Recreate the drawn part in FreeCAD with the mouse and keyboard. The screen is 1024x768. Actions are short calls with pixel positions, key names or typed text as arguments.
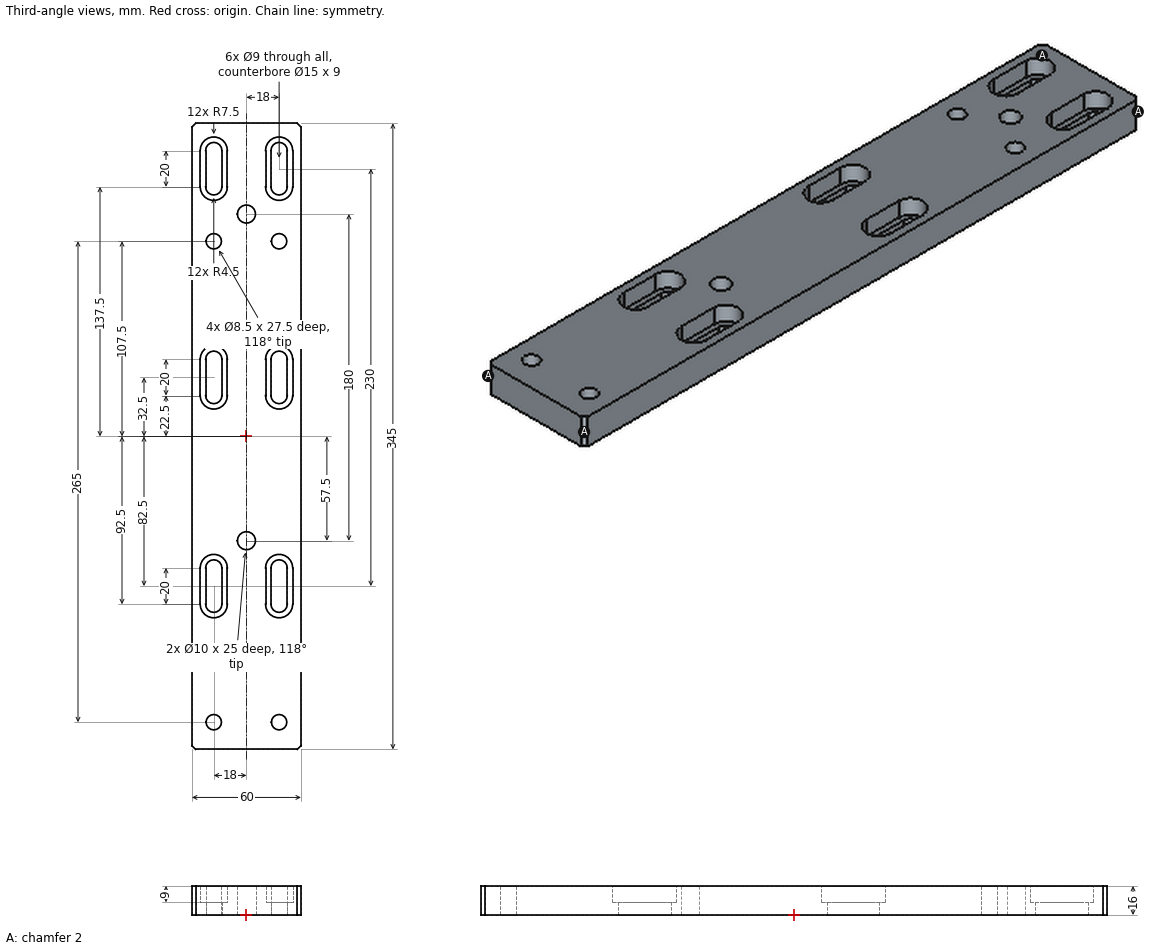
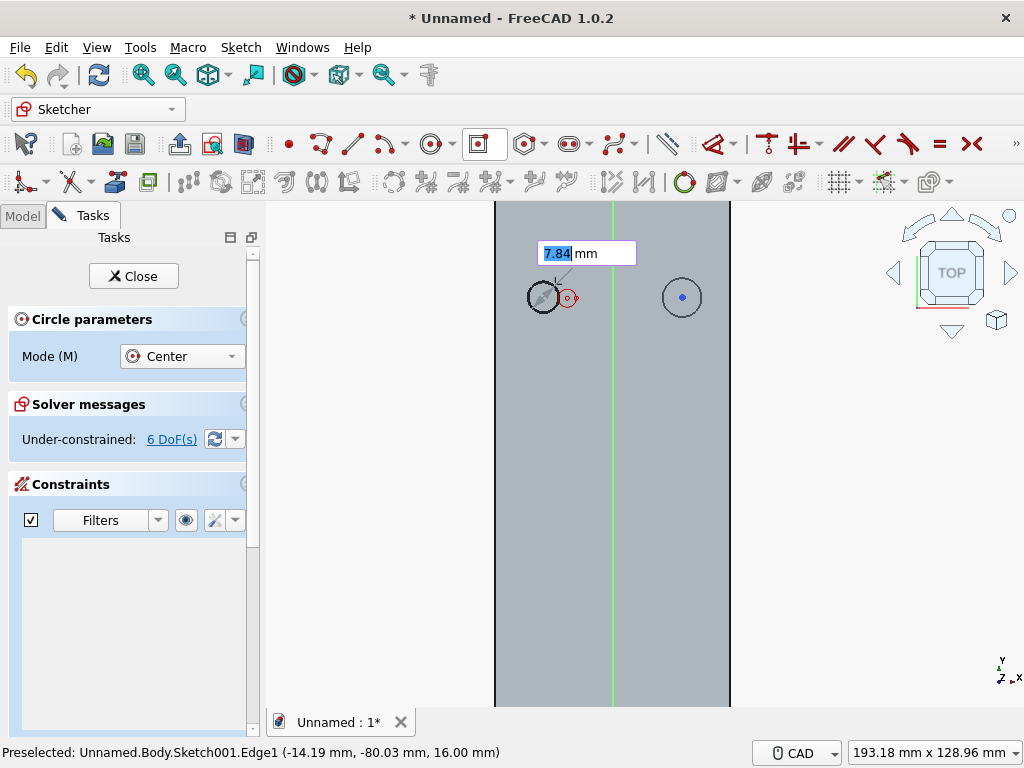
click(555, 283)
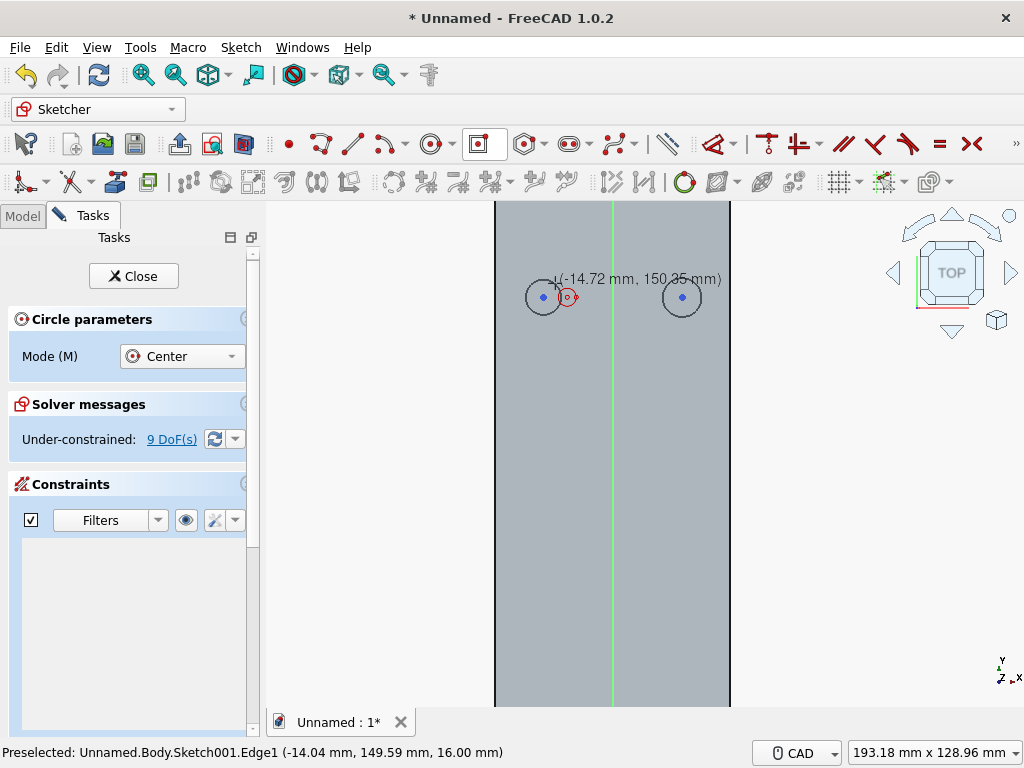
scroll(555, 284, down, 5)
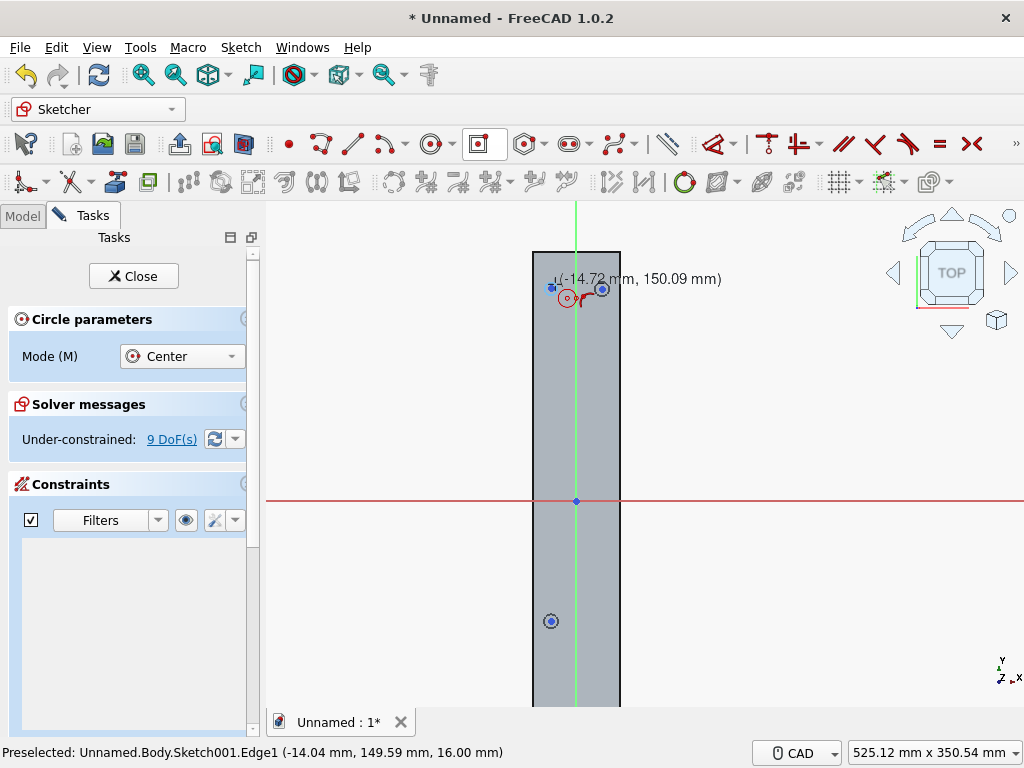
scroll(602, 620, up, 7)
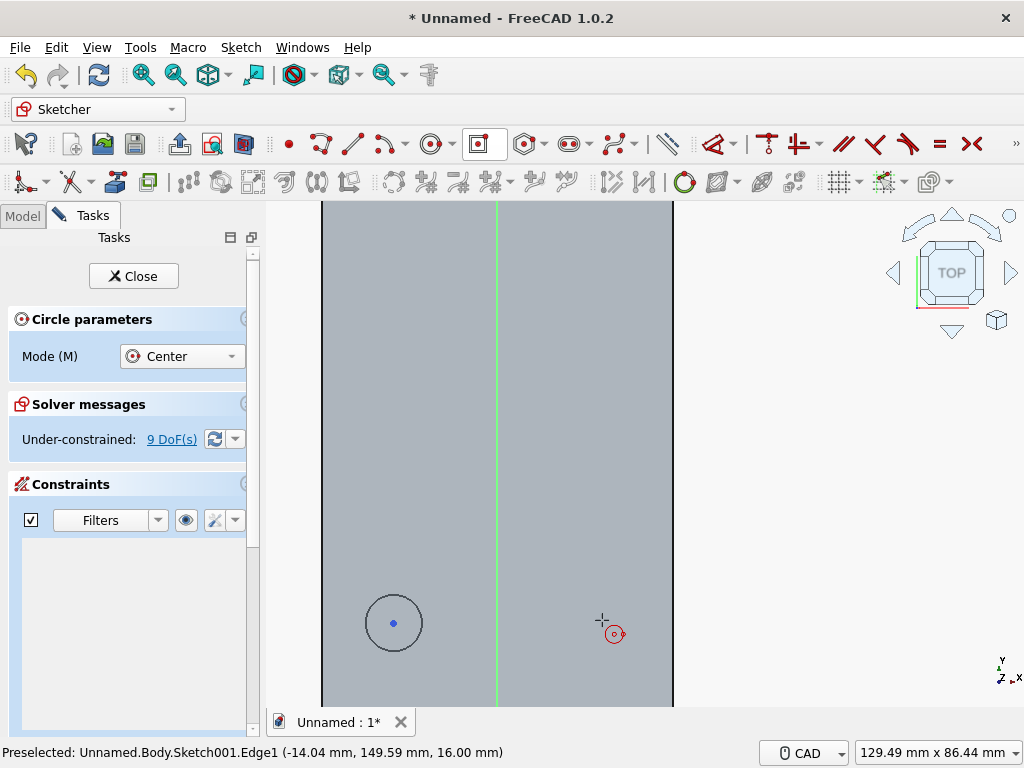
scroll(602, 621, down, 7)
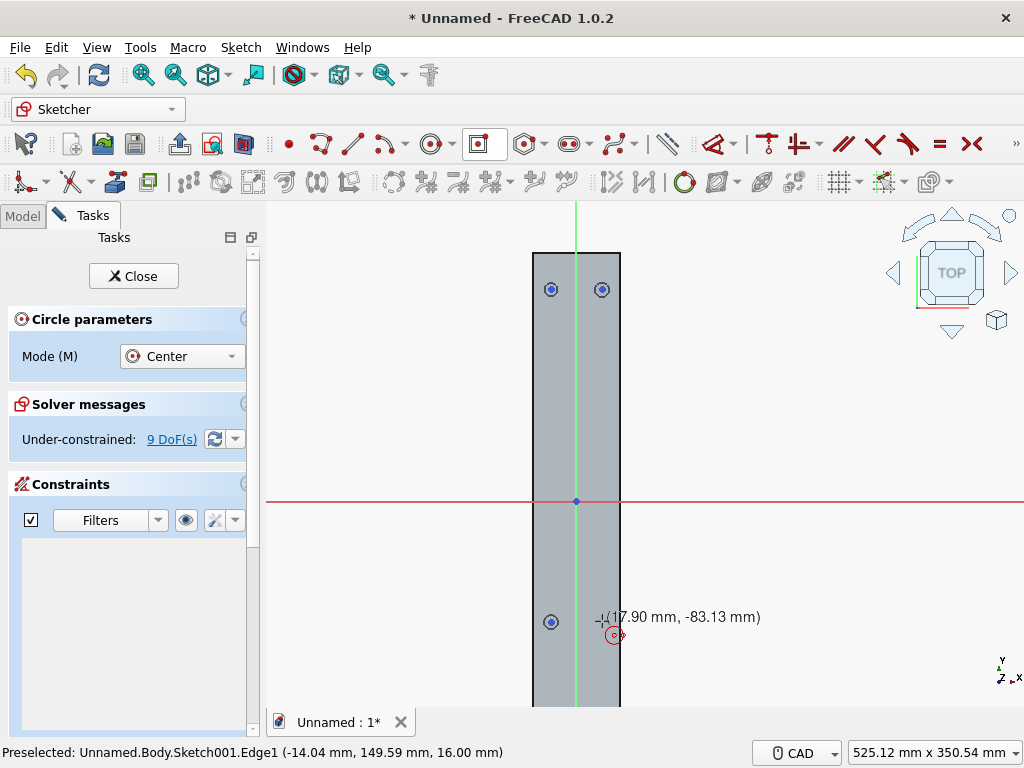
click(602, 621)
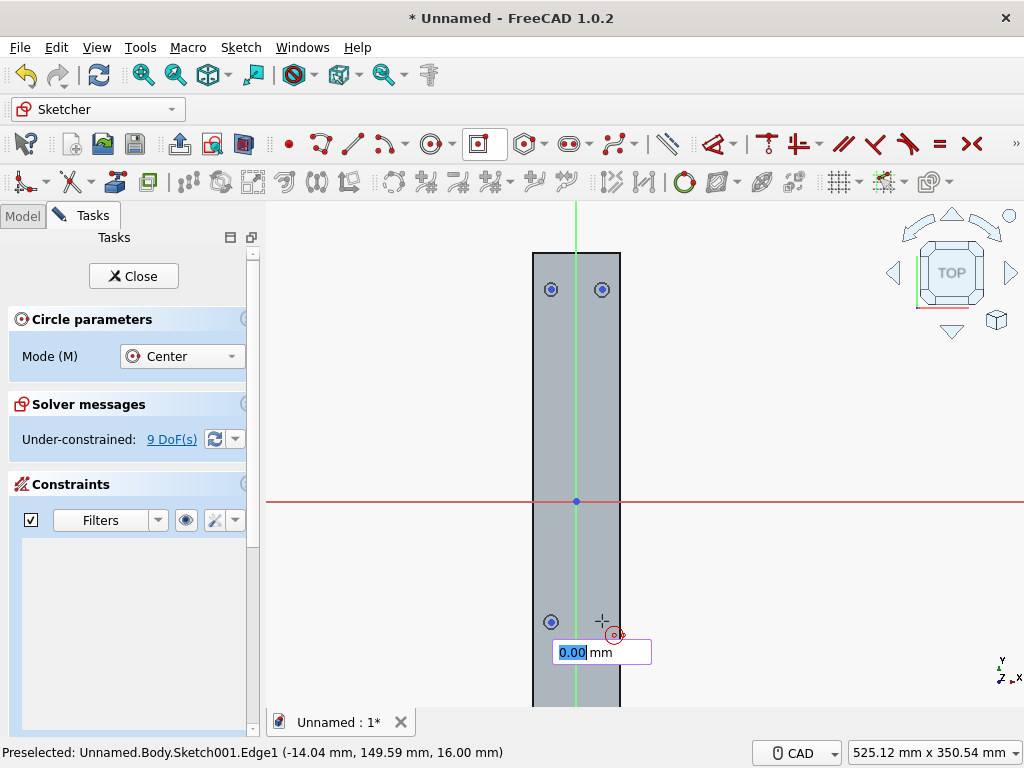
scroll(607, 616, up, 5)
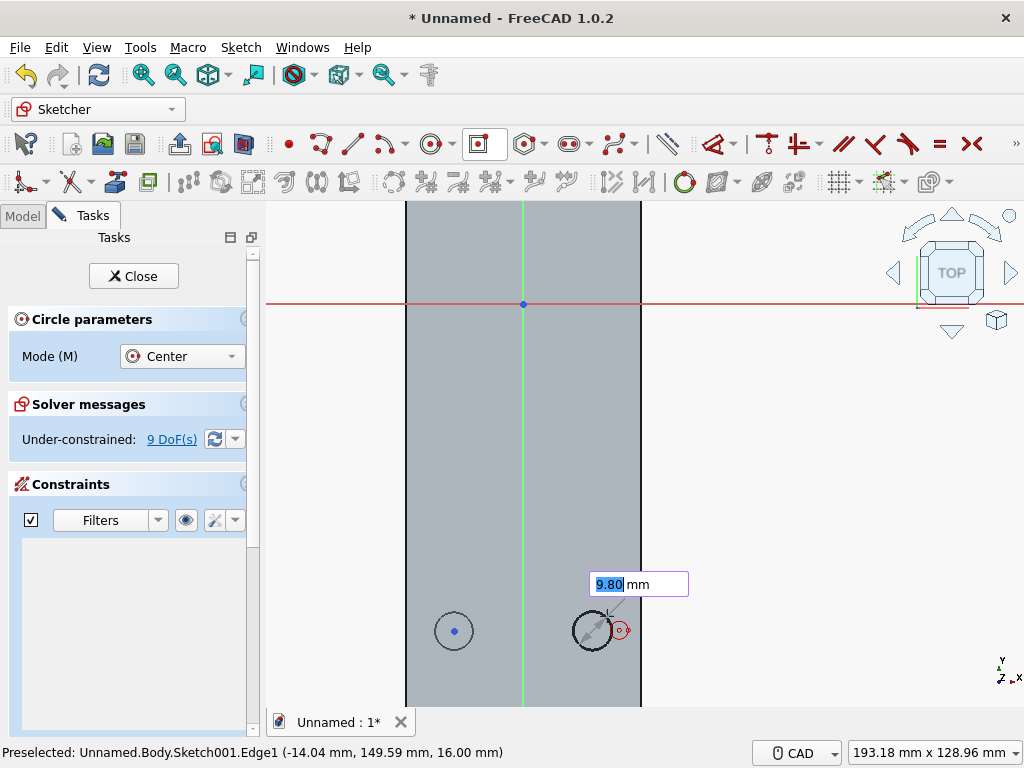
click(606, 616)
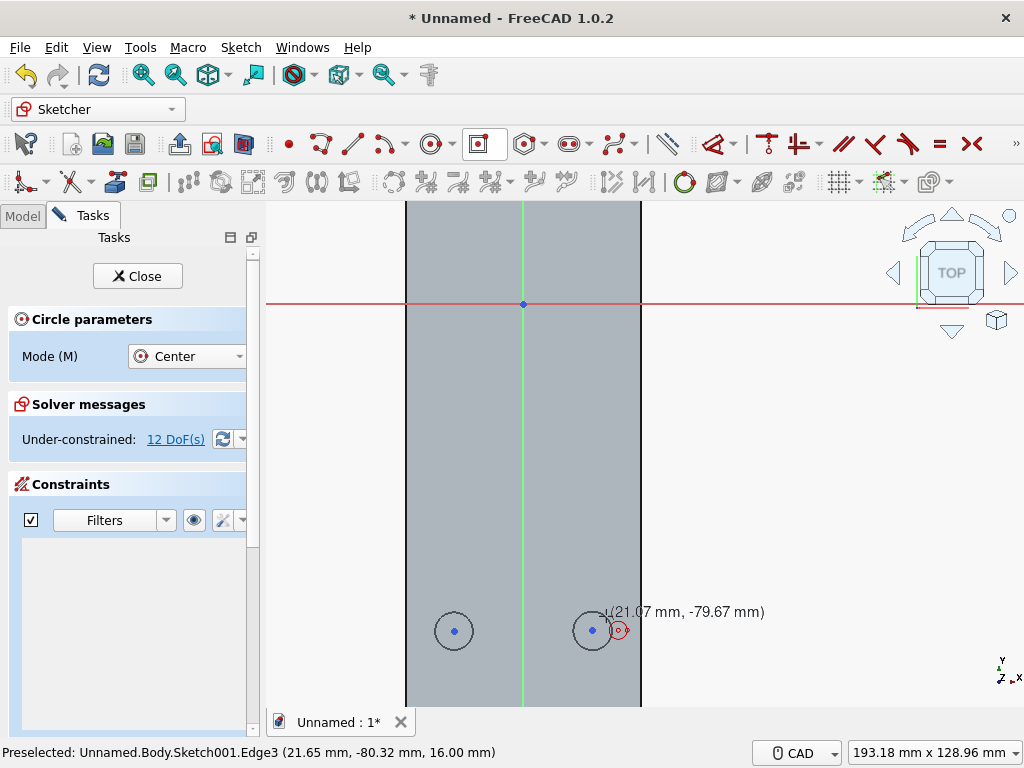
scroll(607, 615, down, 5)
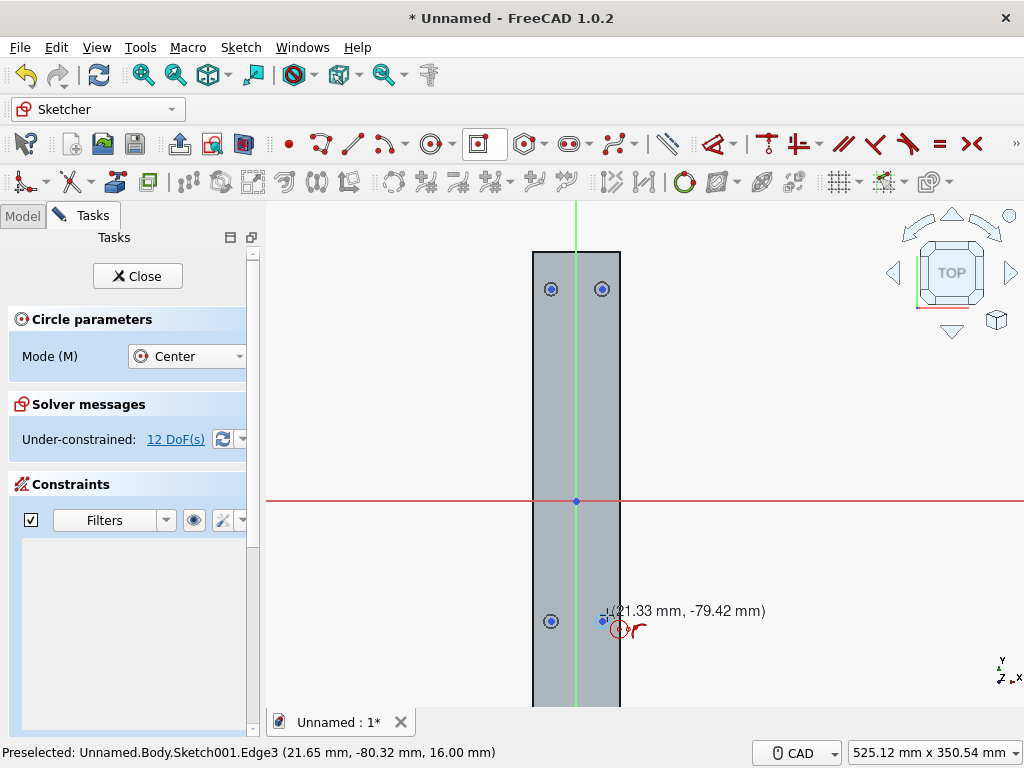
scroll(551, 454, up, 7)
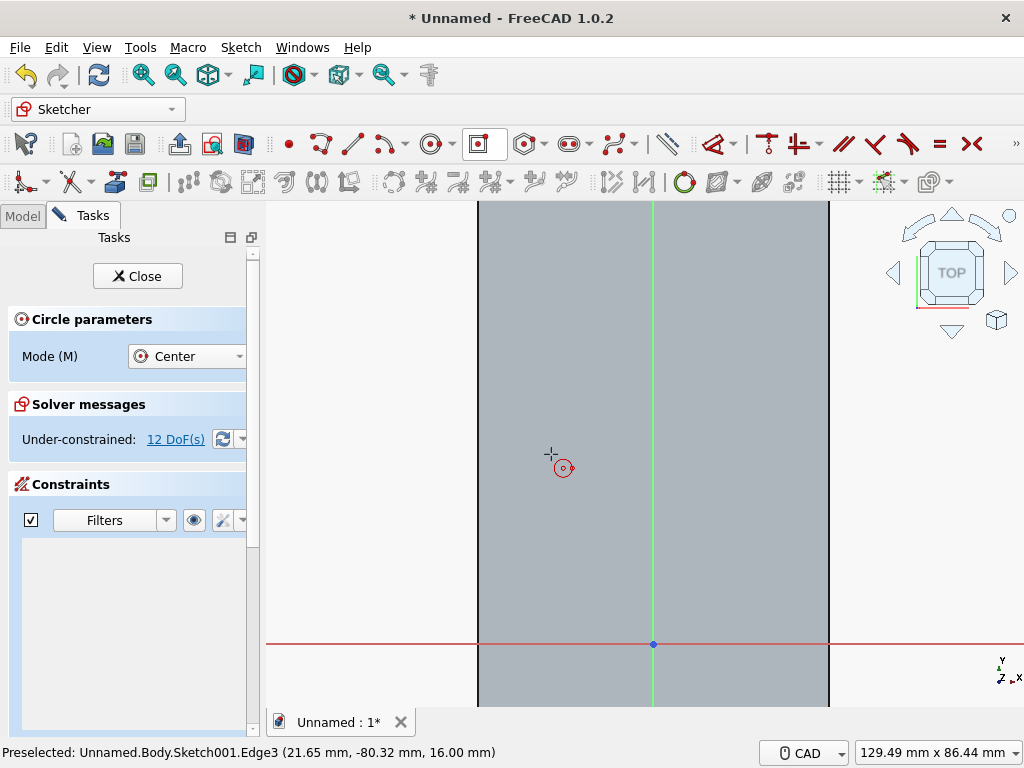
scroll(551, 454, down, 7)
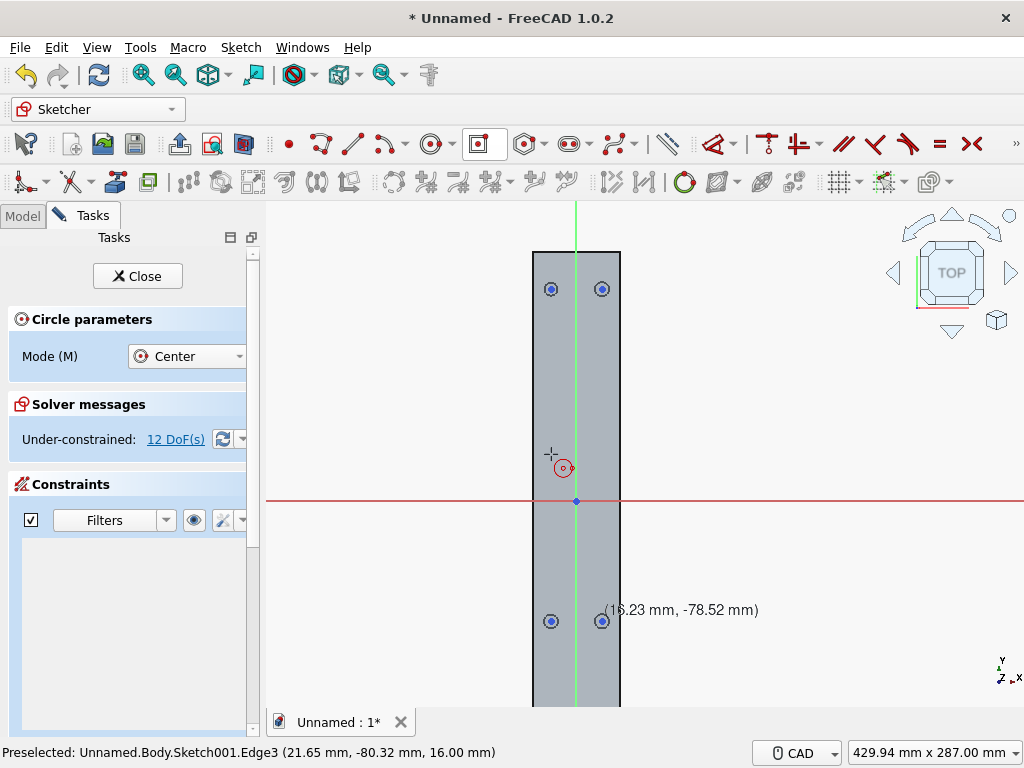
click(551, 454)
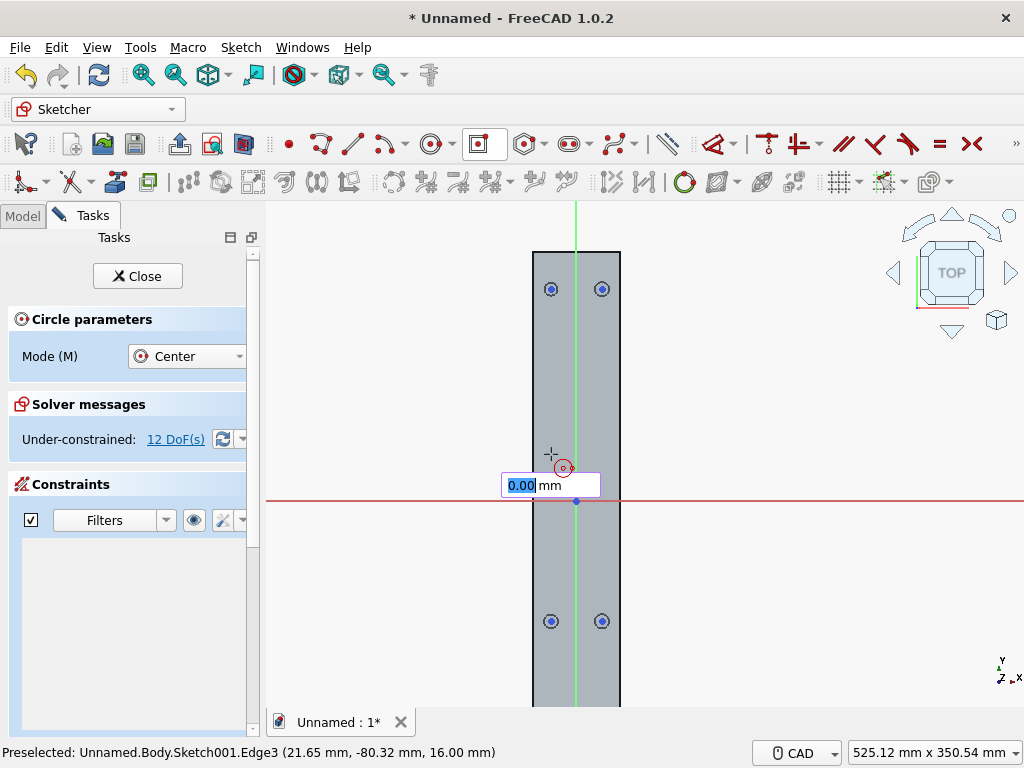
scroll(555, 450, up, 5)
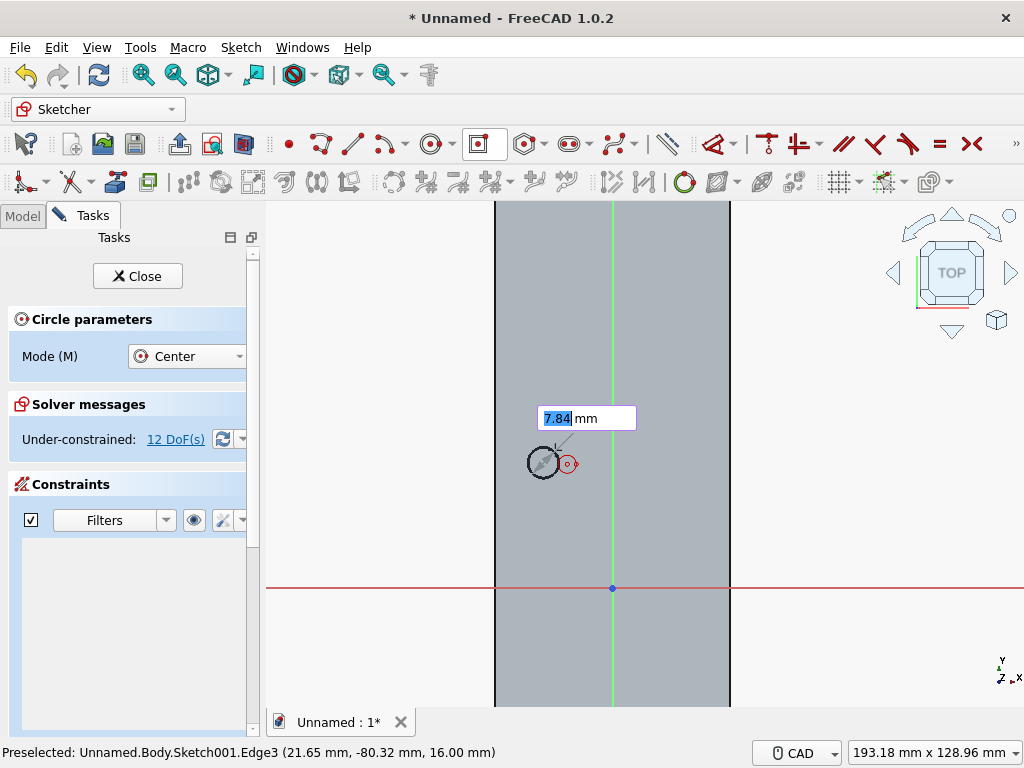
click(555, 448)